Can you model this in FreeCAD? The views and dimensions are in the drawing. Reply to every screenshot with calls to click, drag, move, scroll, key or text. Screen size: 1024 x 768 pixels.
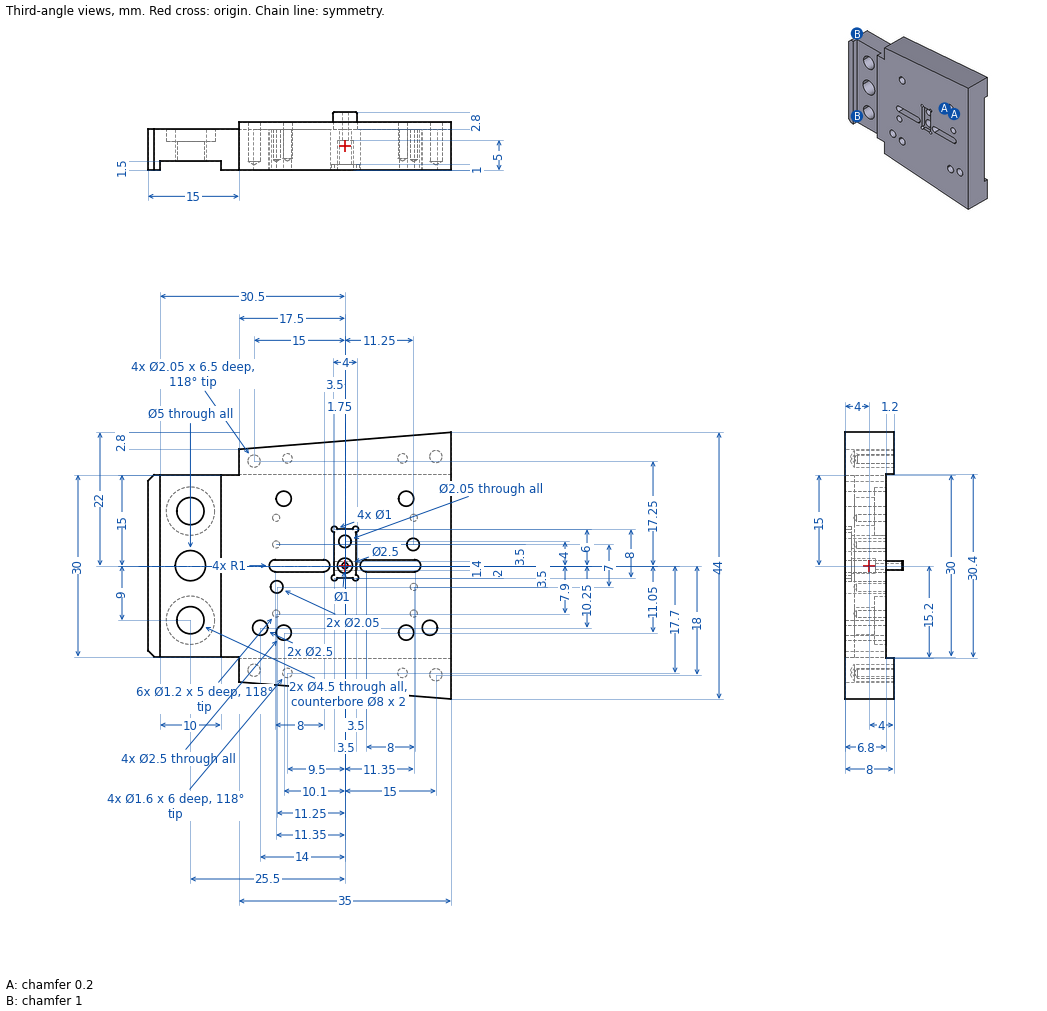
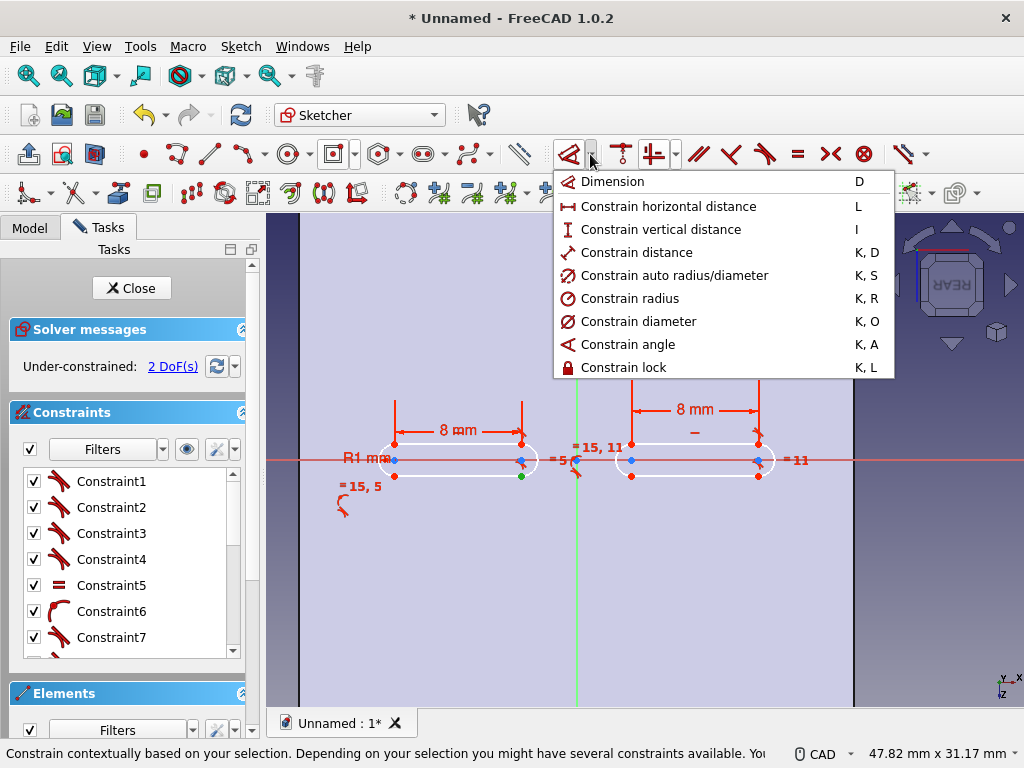
click(724, 206)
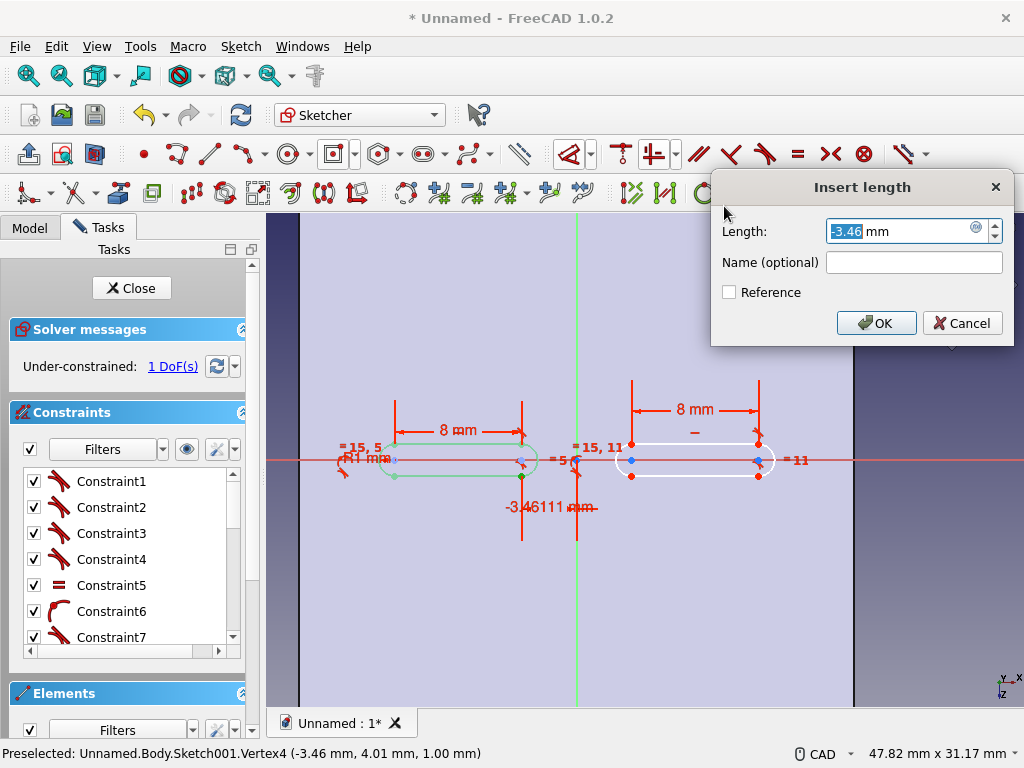
text(-3.5)
key(Return)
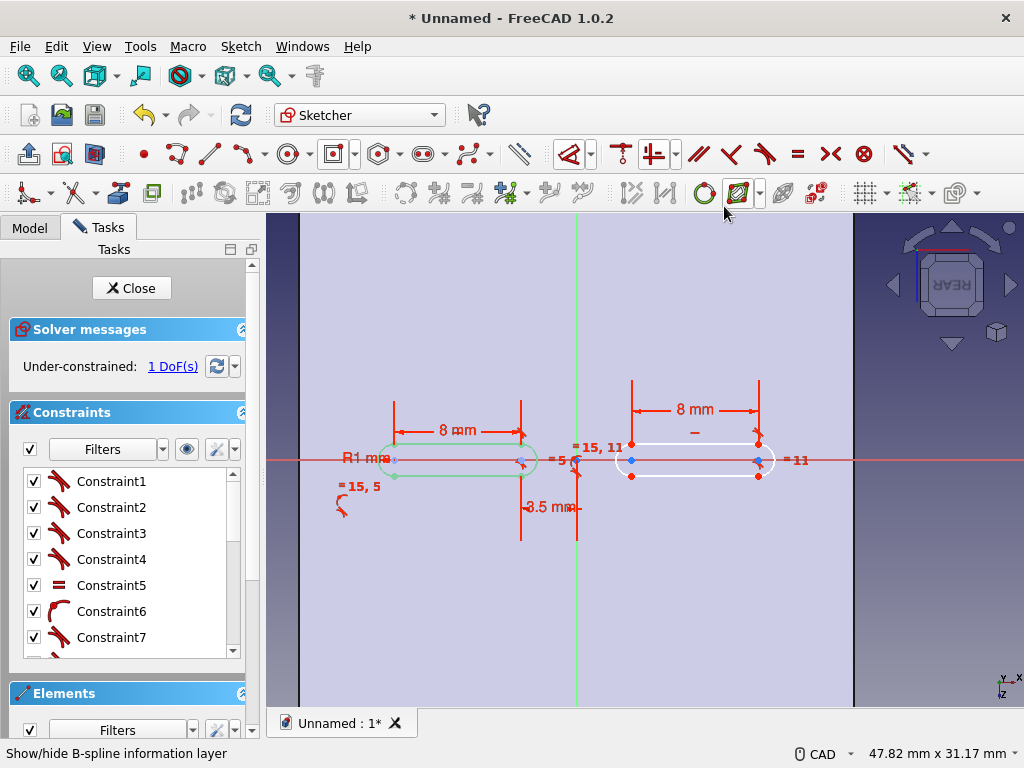
click(632, 444)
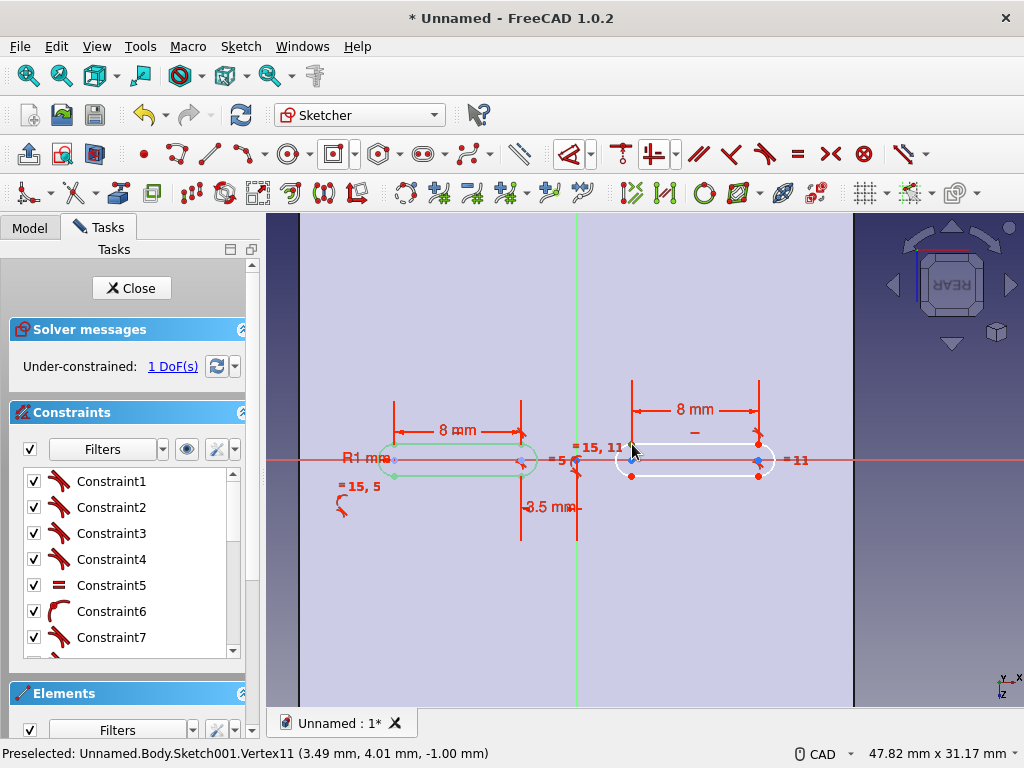
click(590, 154)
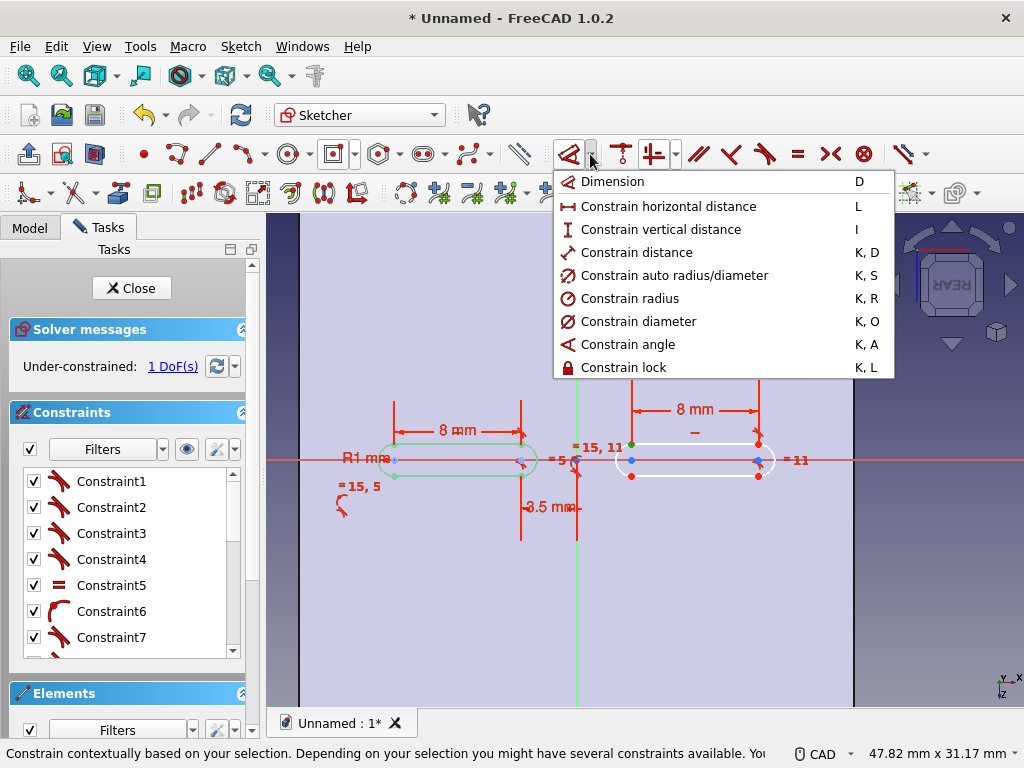
click(724, 206)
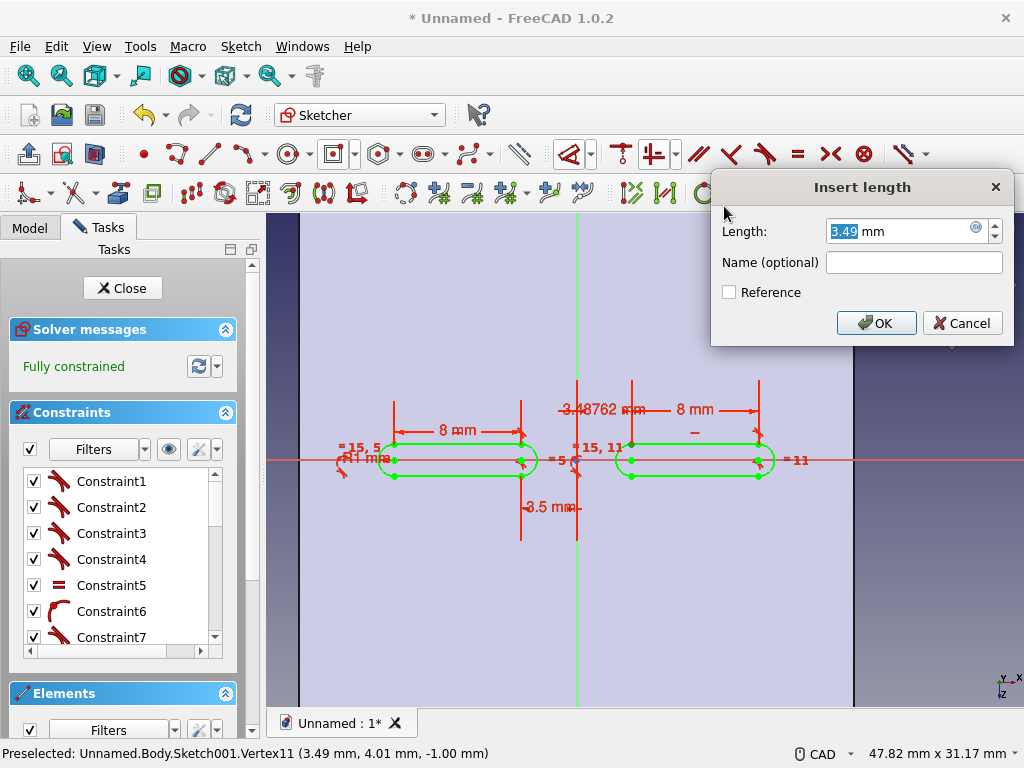
text(3.5)
key(Return)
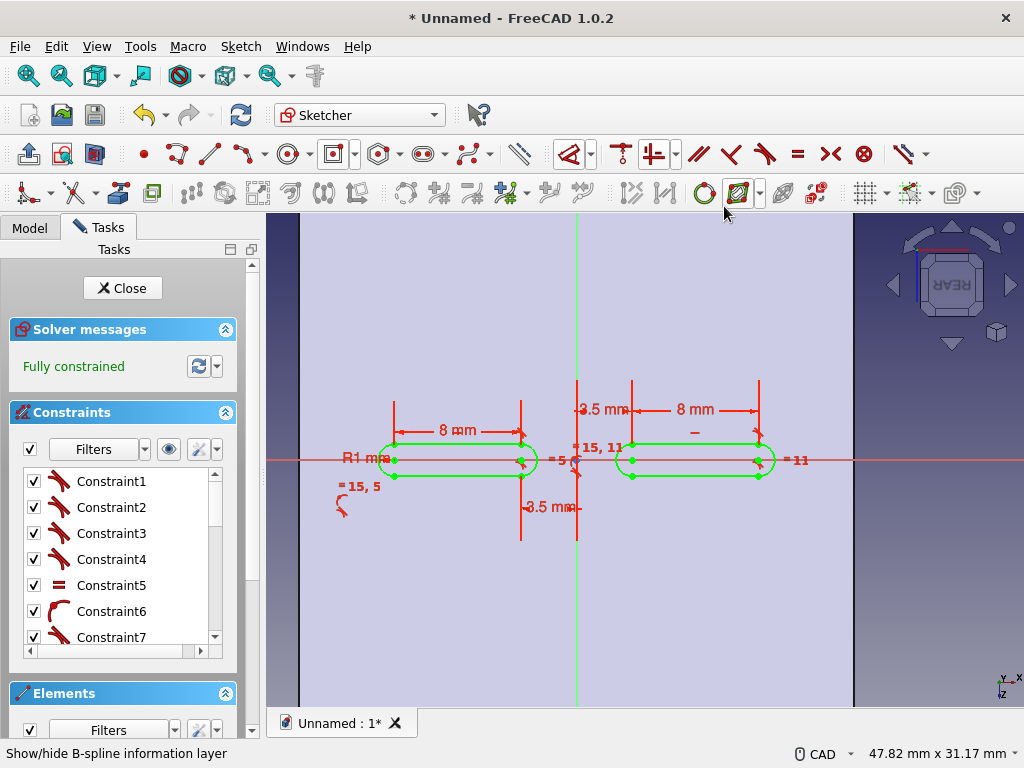
click(123, 288)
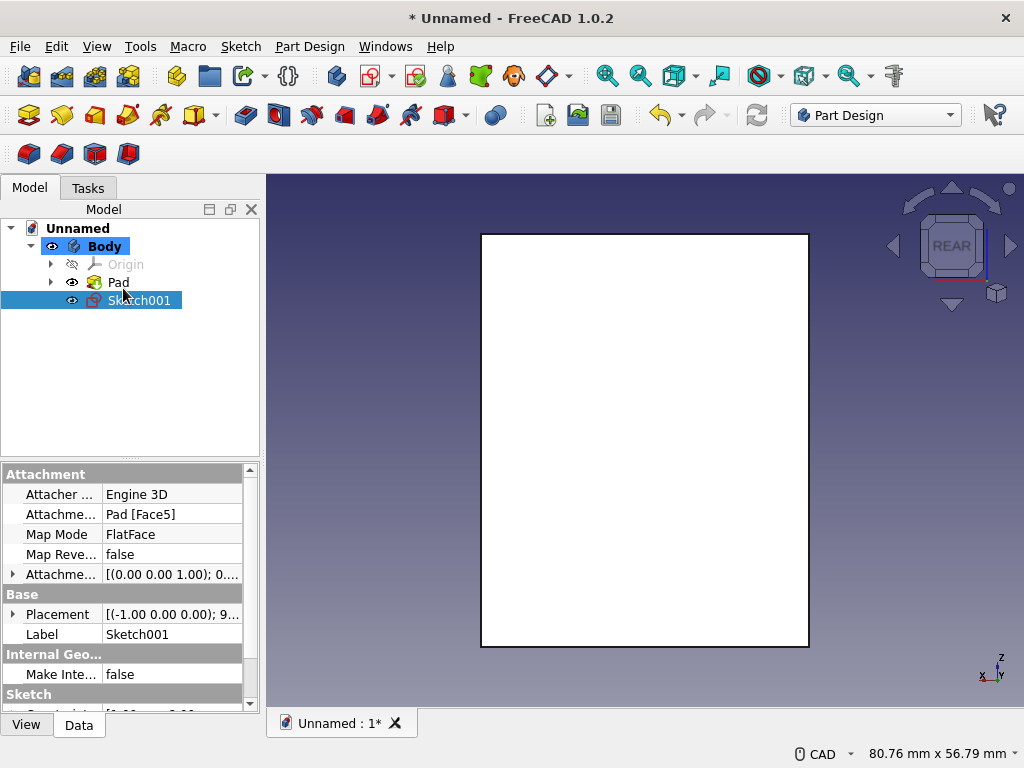
click(246, 116)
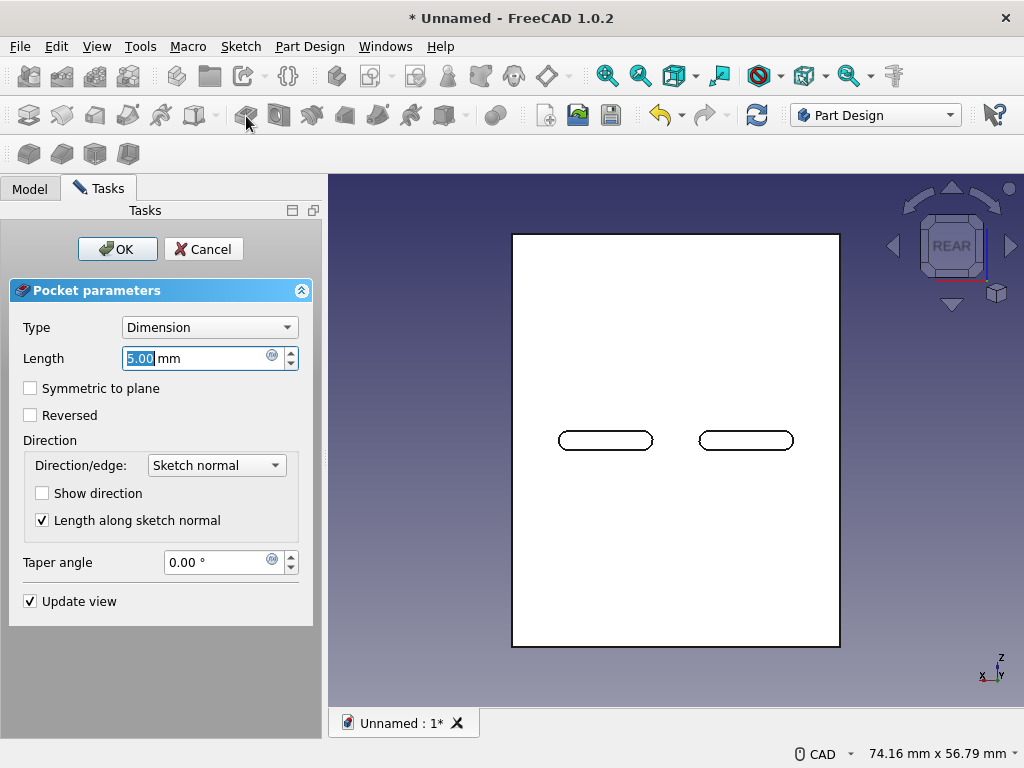
click(210, 328)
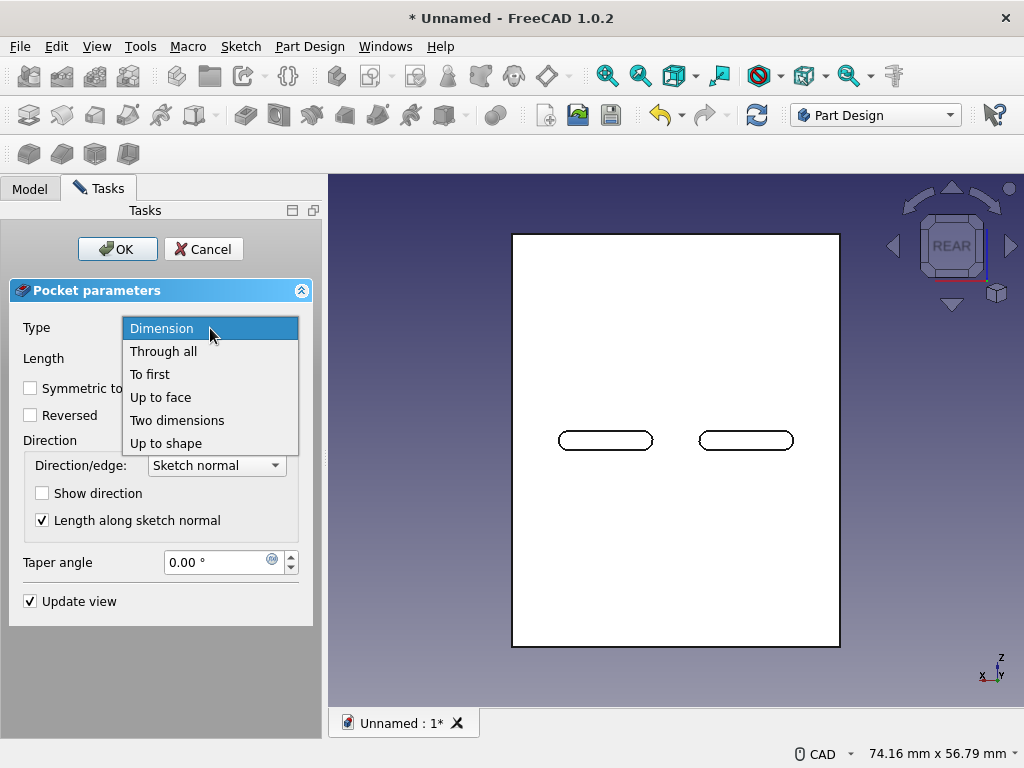
click(208, 352)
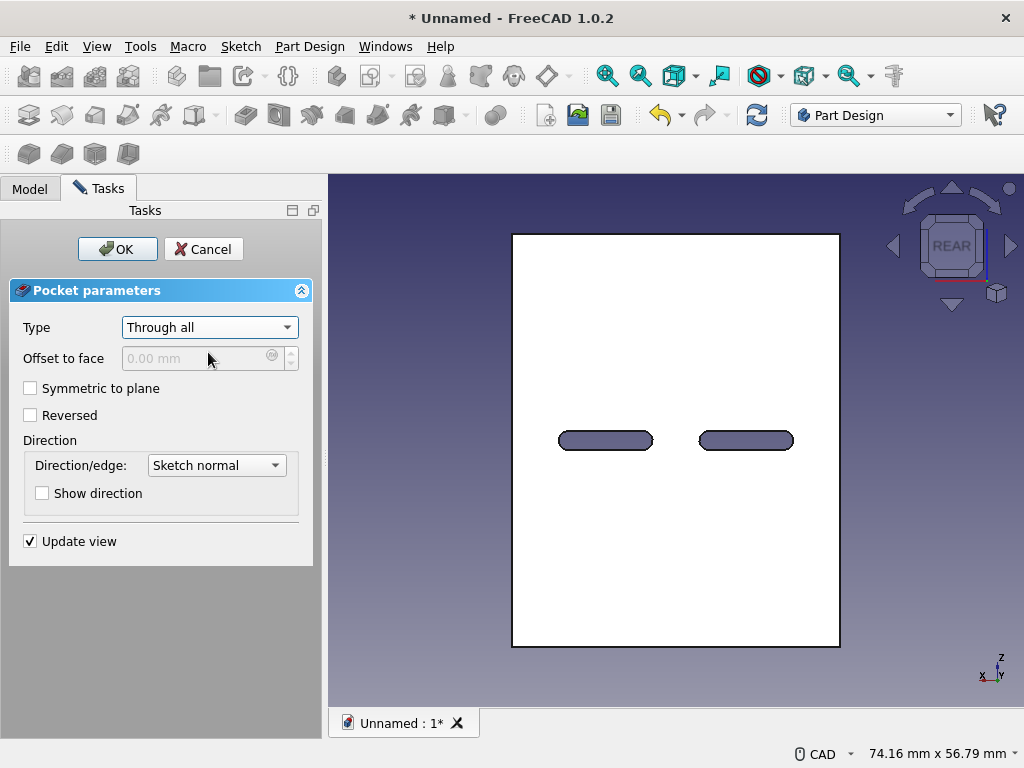
click(118, 249)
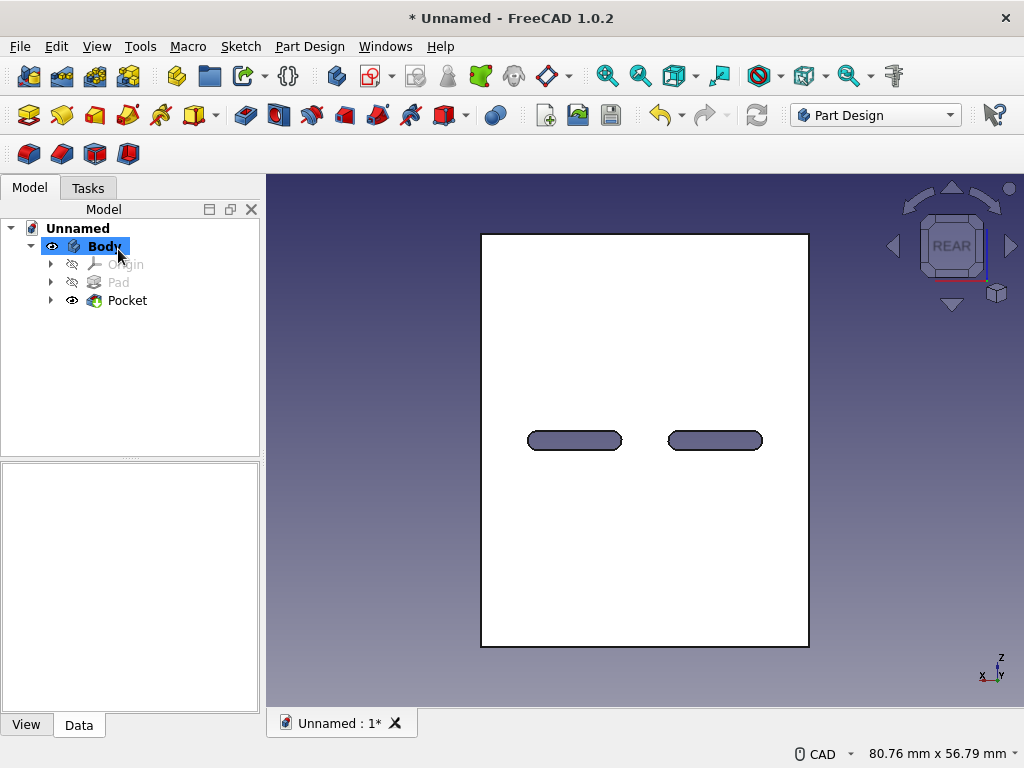
key(0)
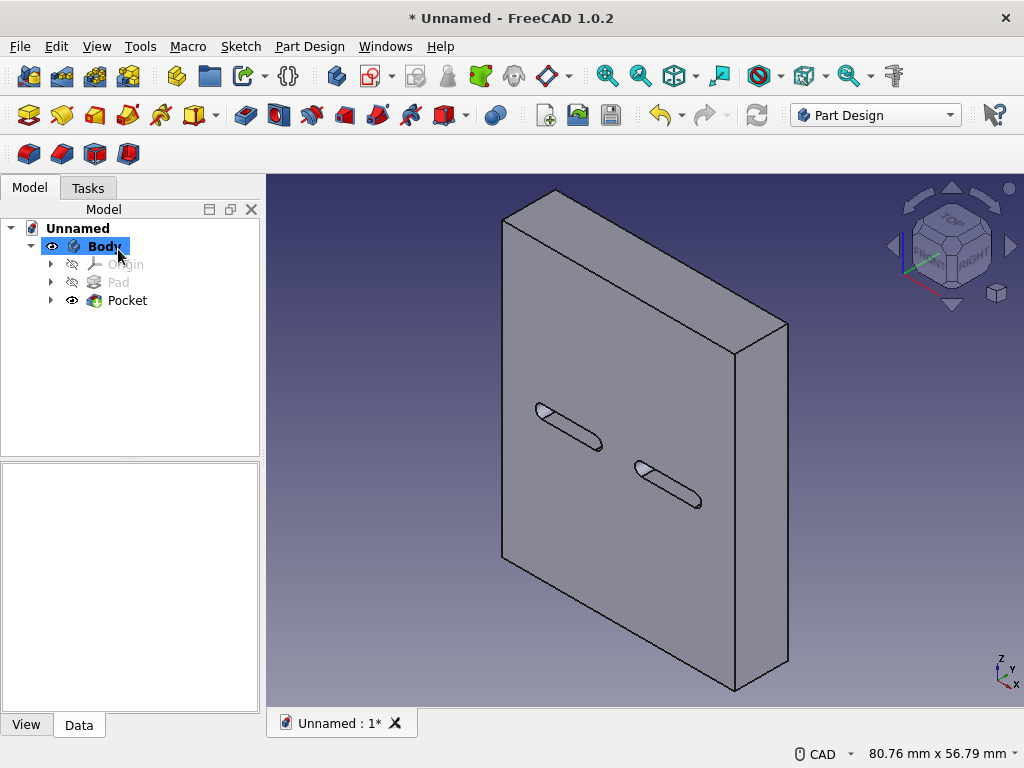
click(761, 410)